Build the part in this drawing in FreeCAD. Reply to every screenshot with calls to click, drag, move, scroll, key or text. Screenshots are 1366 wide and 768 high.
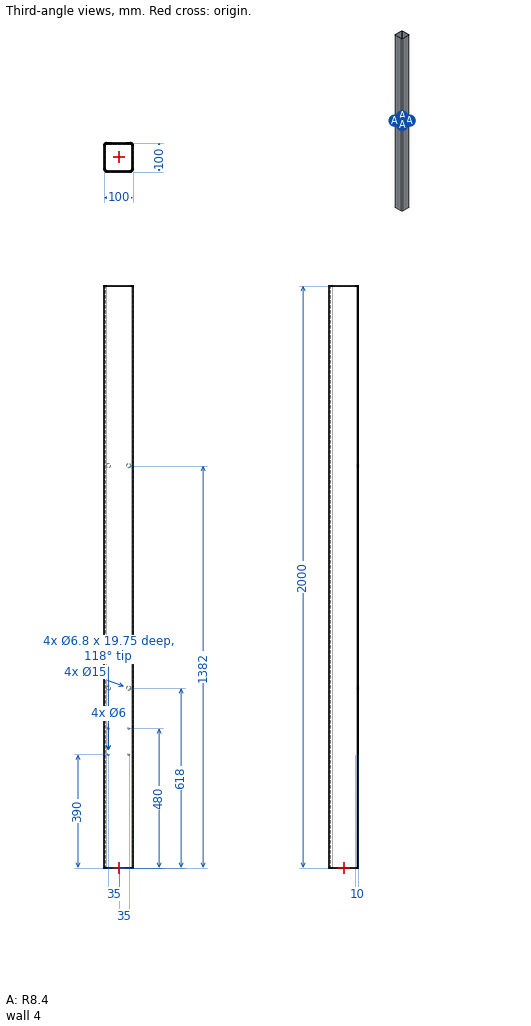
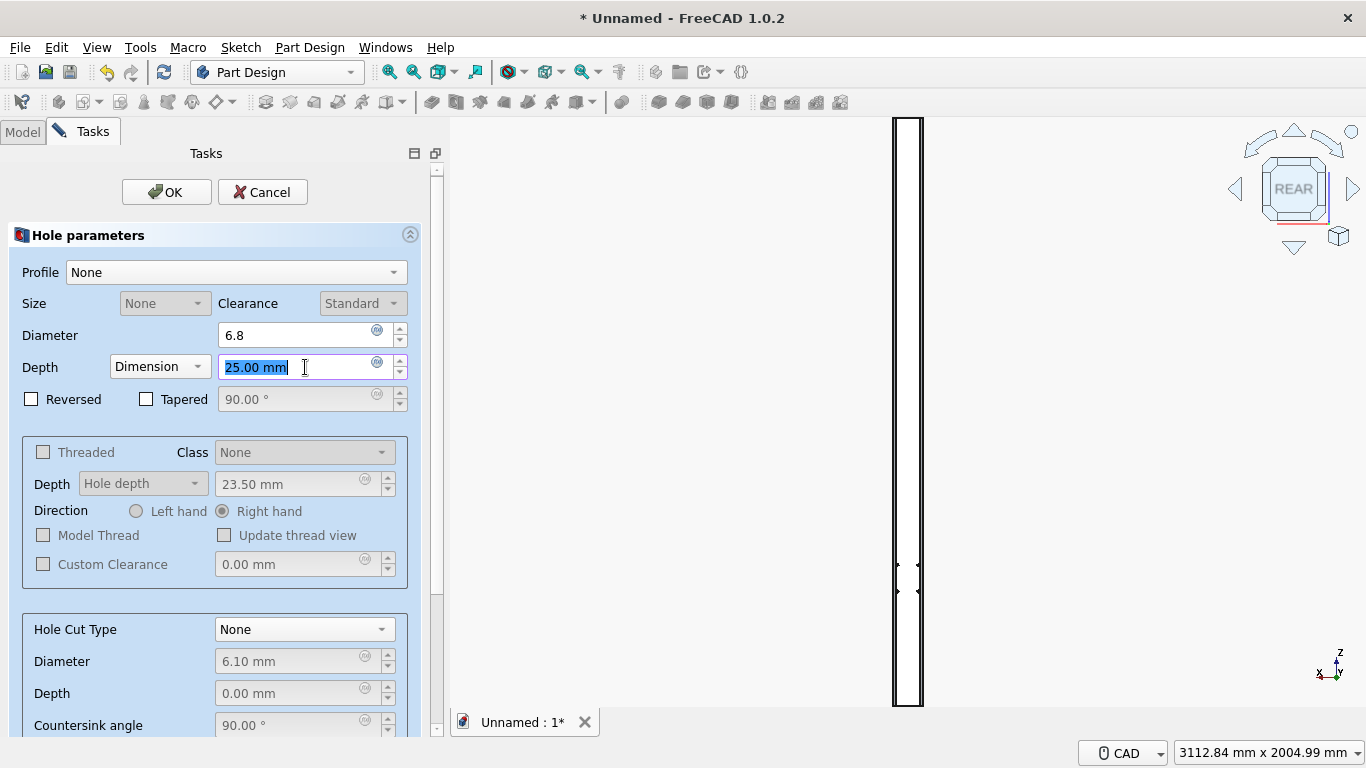
text(19.75)
key(Tab)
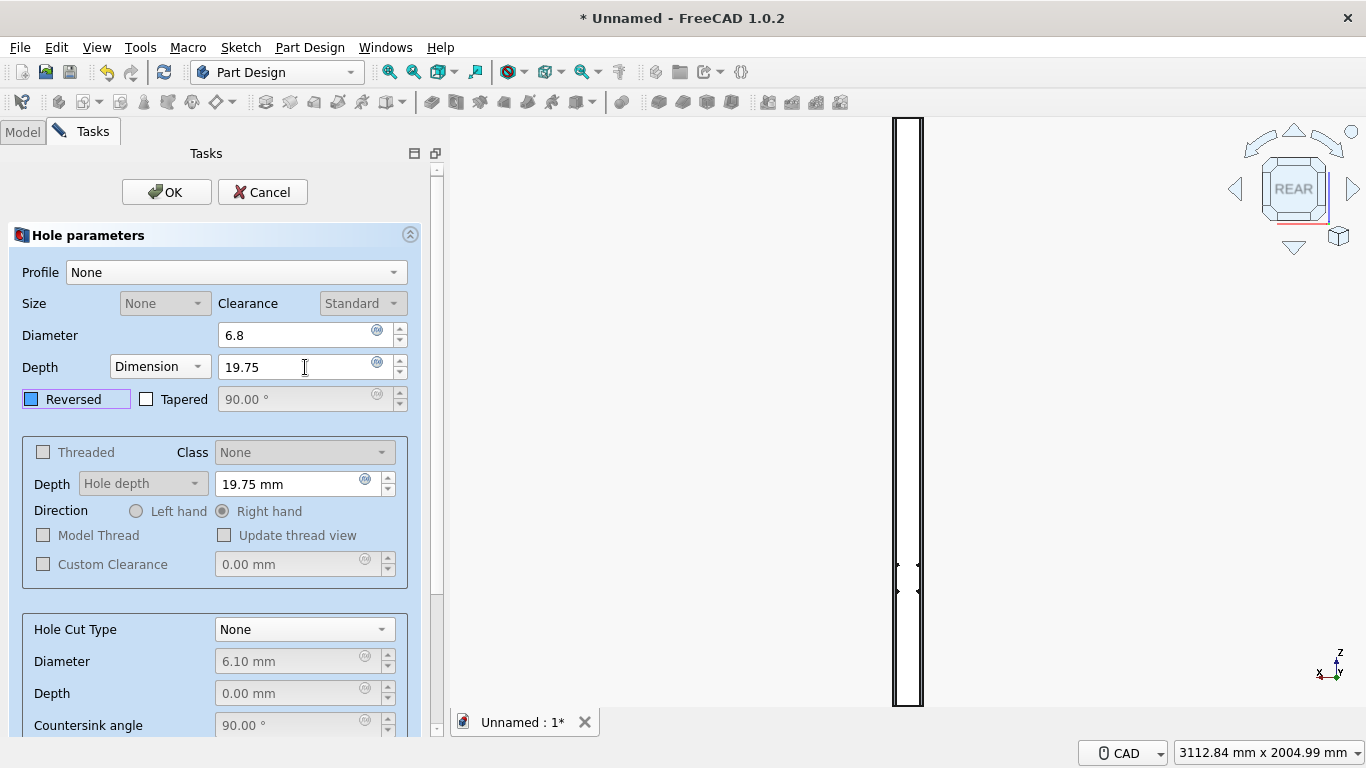
click(167, 192)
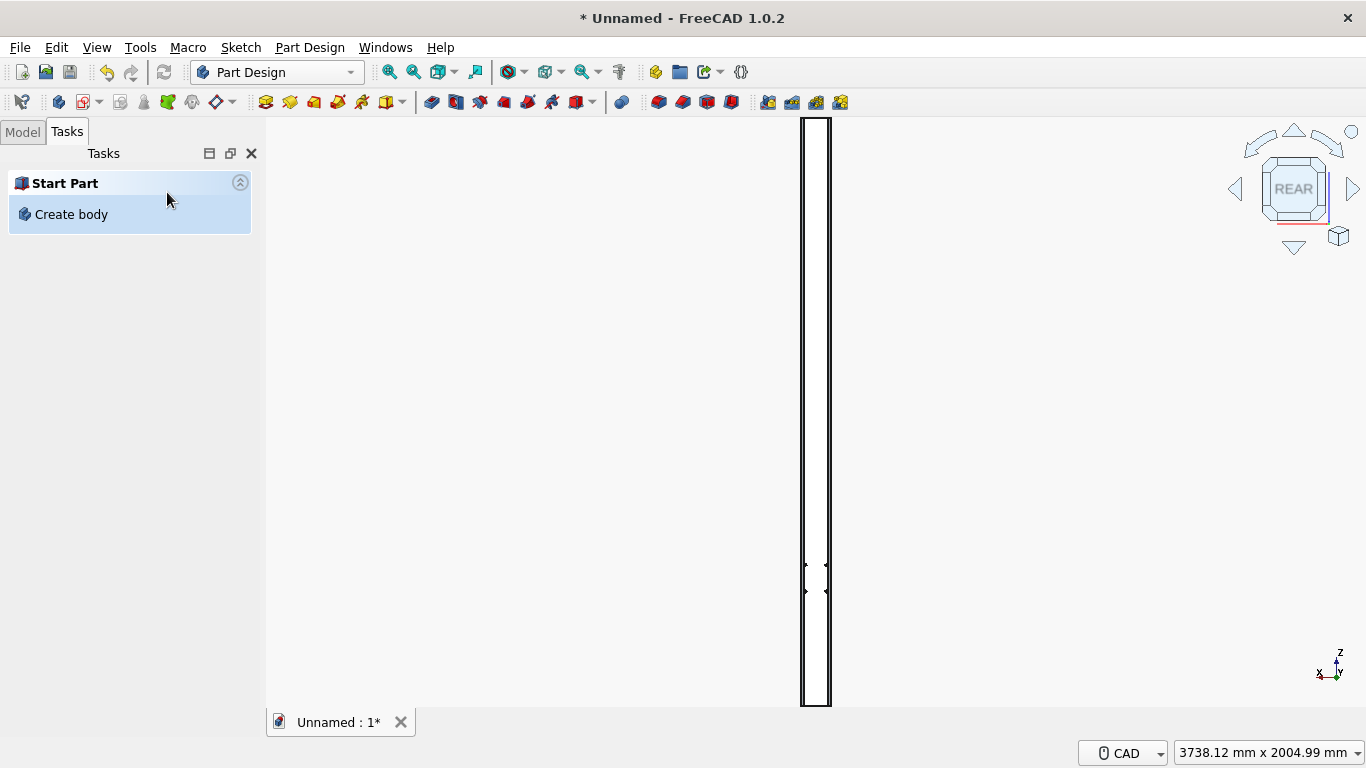
click(816, 159)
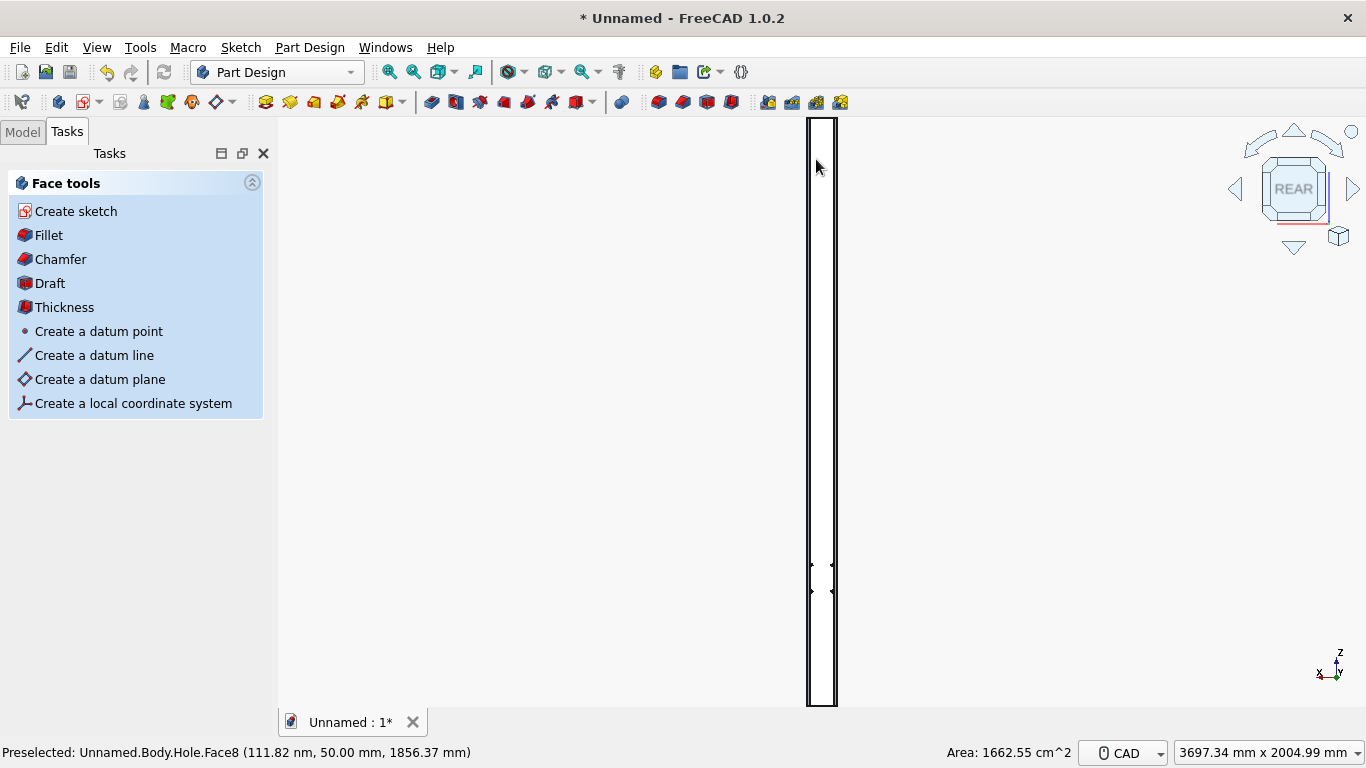
click(84, 102)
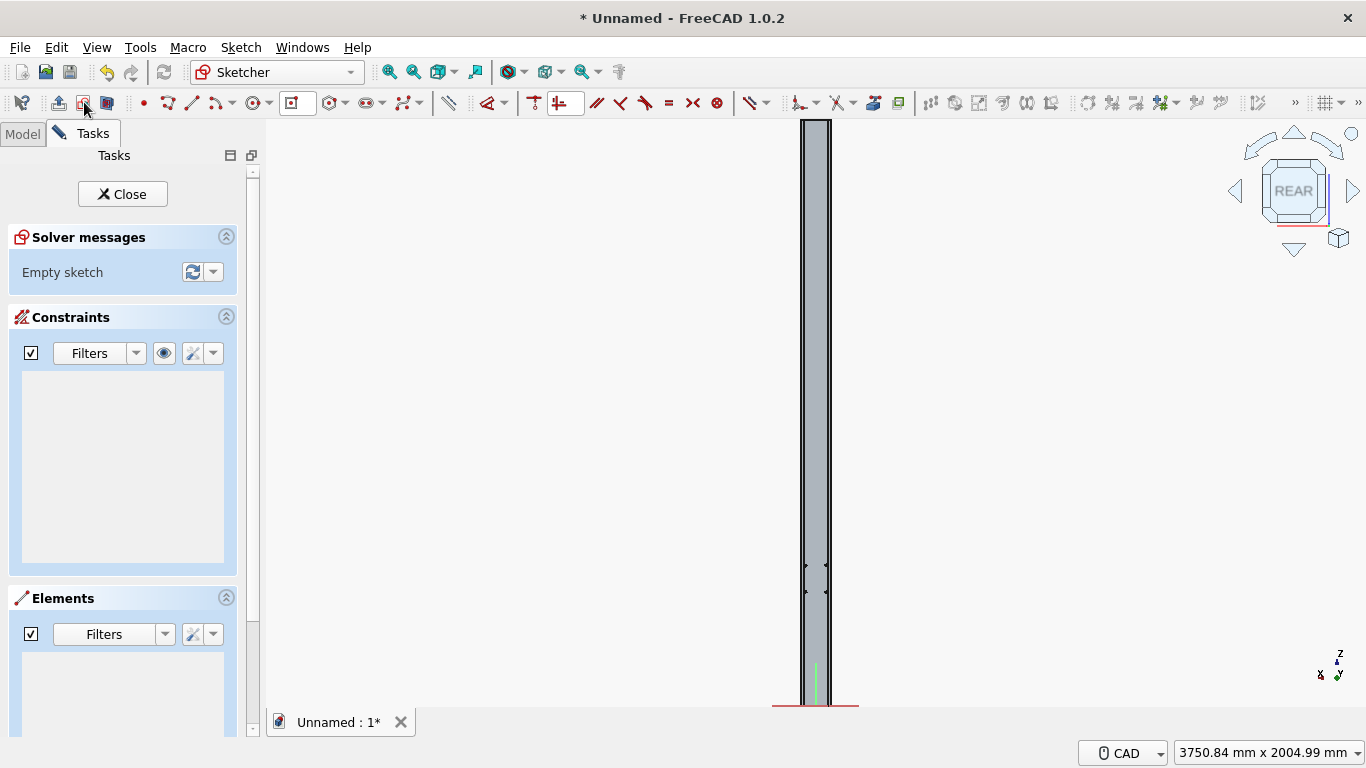
scroll(438, 147, down, 1)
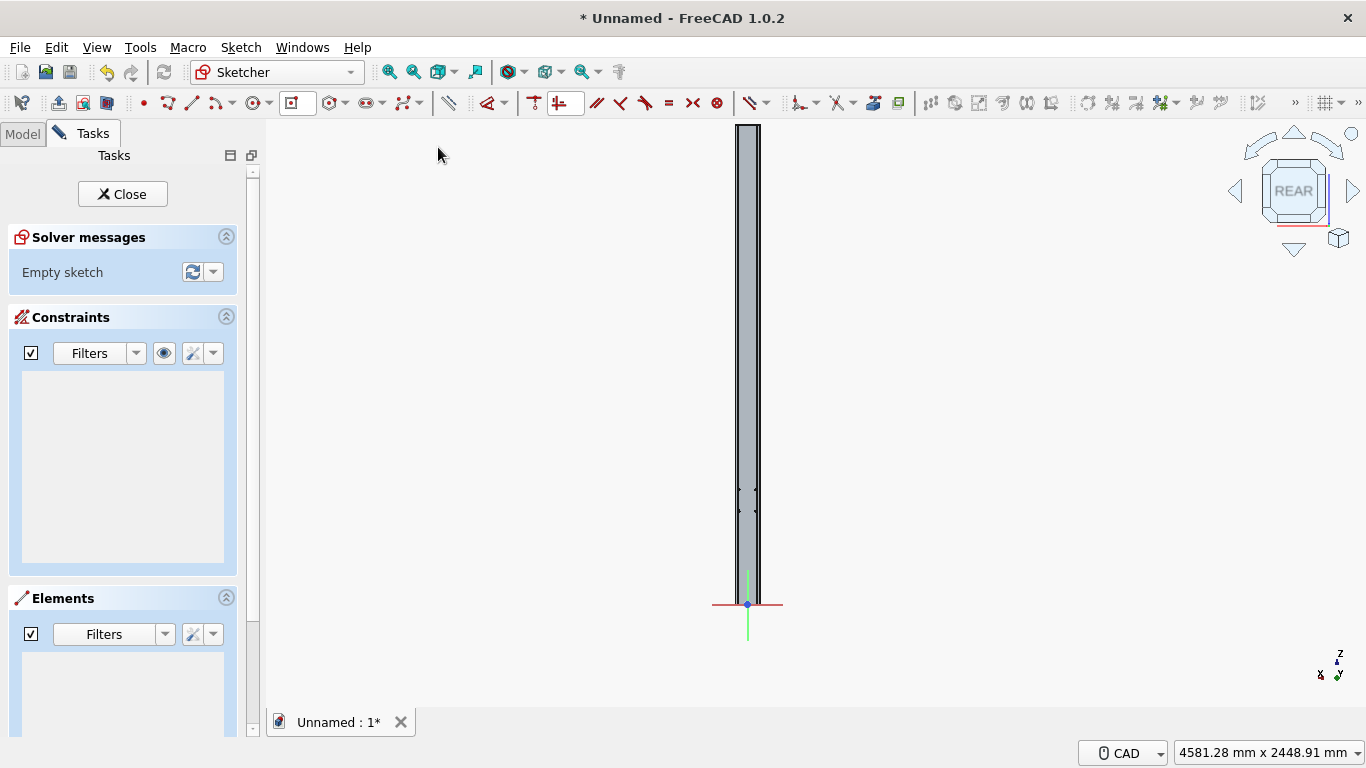
click(254, 104)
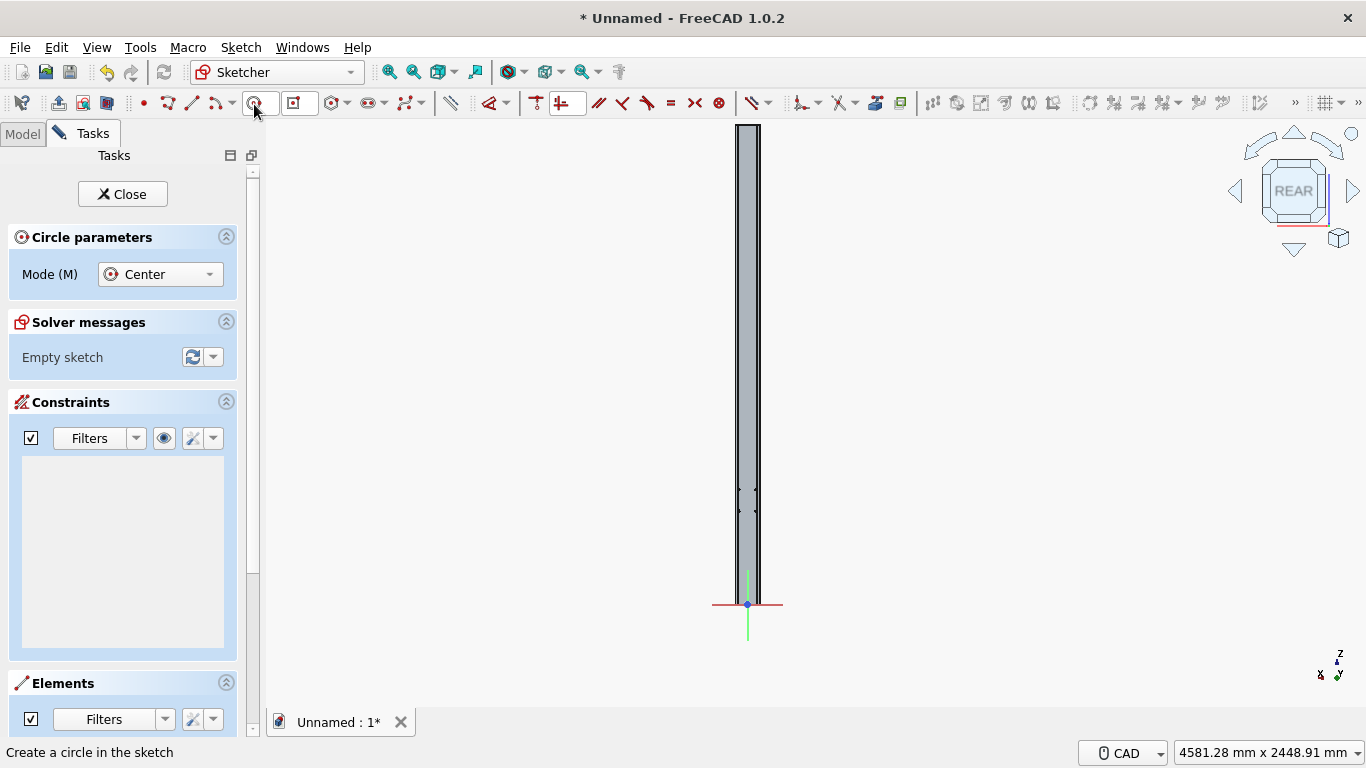
scroll(739, 457, up, 13)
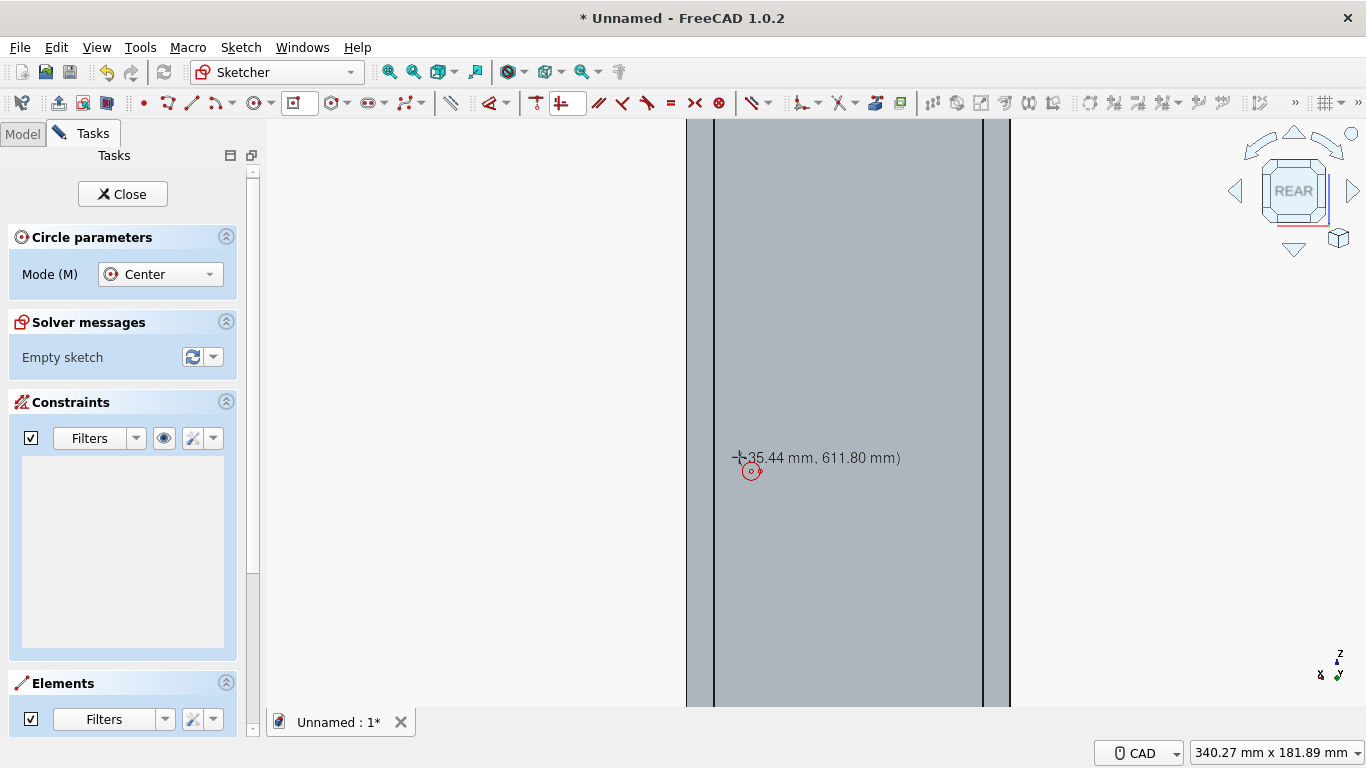
scroll(737, 435, down, 12)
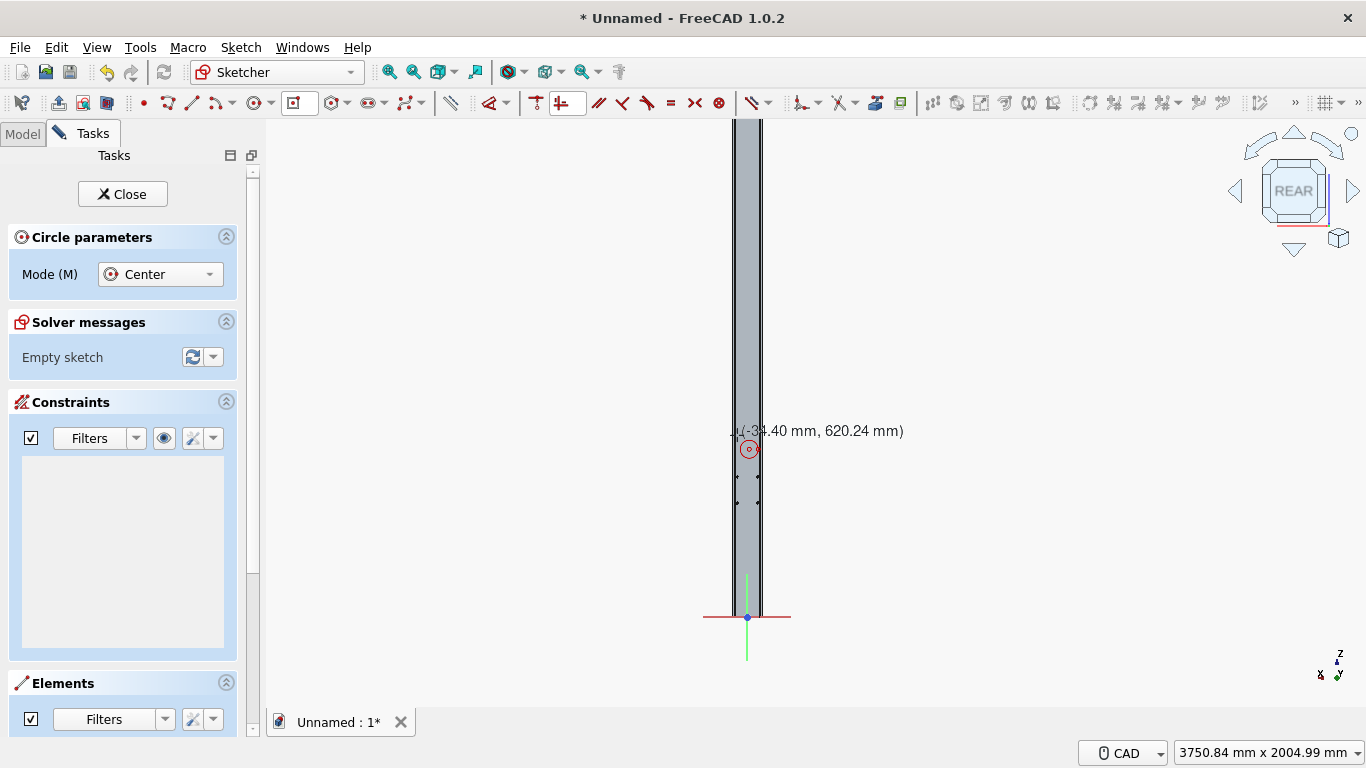
scroll(737, 436, up, 3)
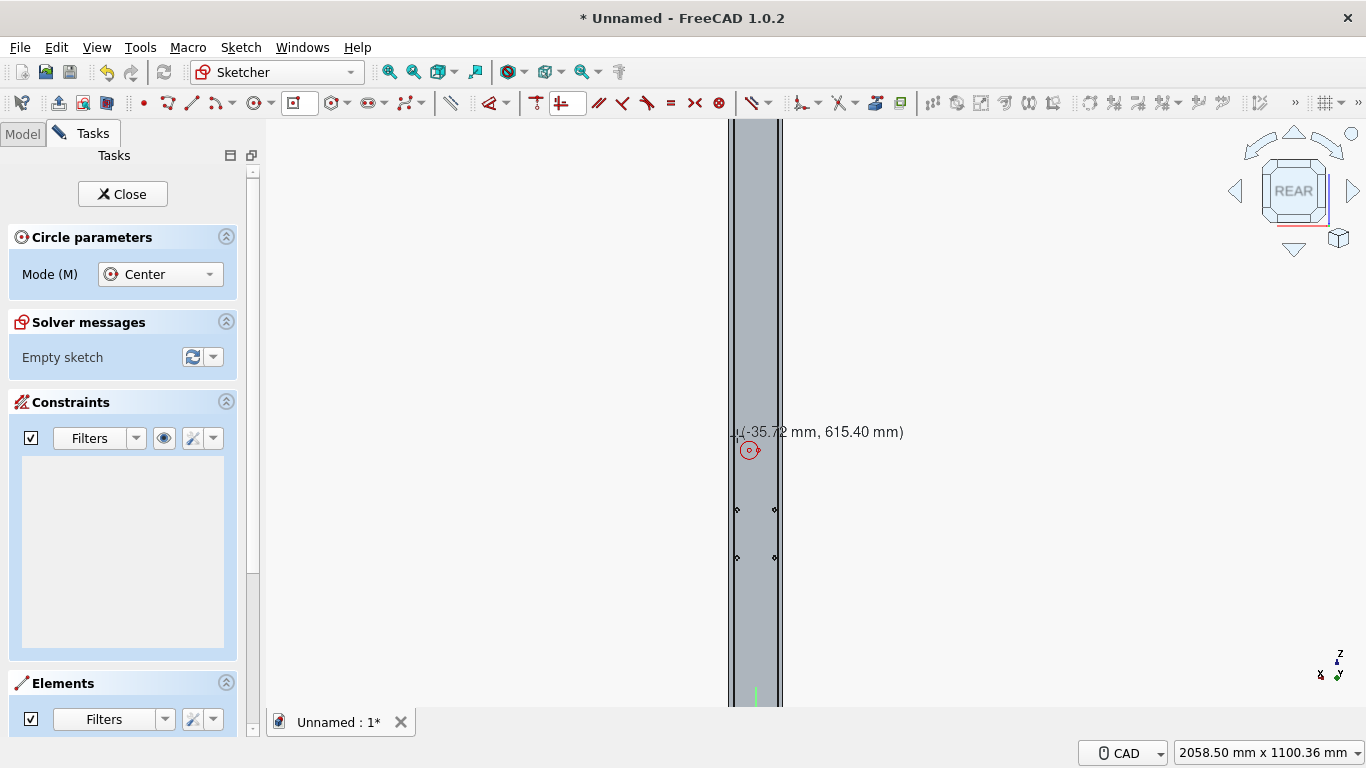
click(737, 436)